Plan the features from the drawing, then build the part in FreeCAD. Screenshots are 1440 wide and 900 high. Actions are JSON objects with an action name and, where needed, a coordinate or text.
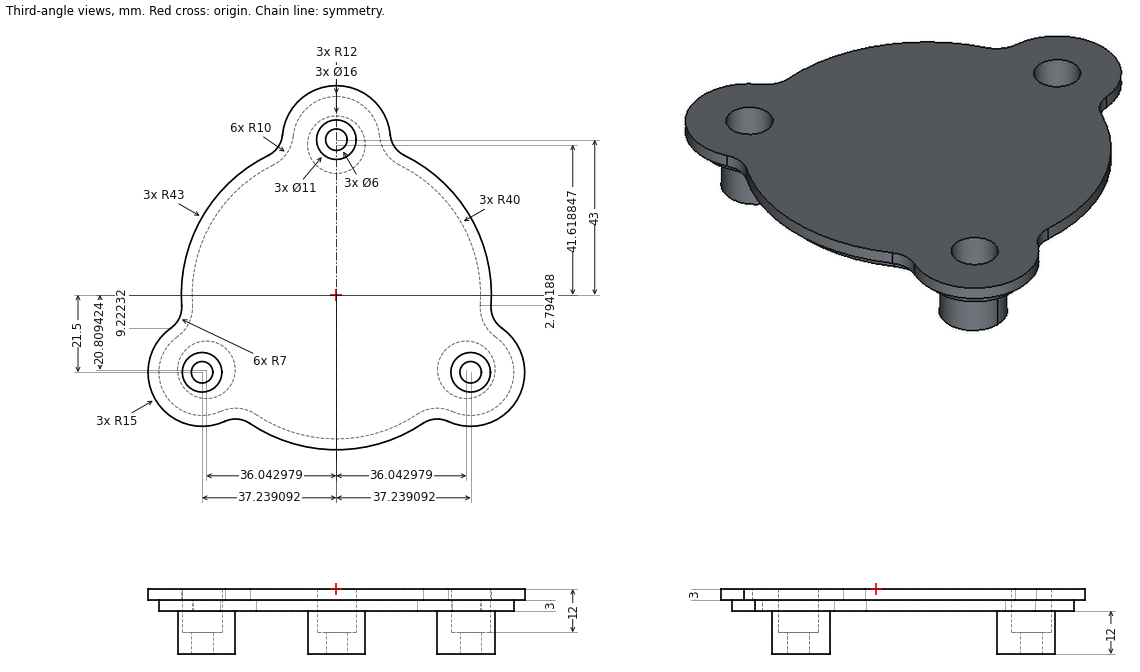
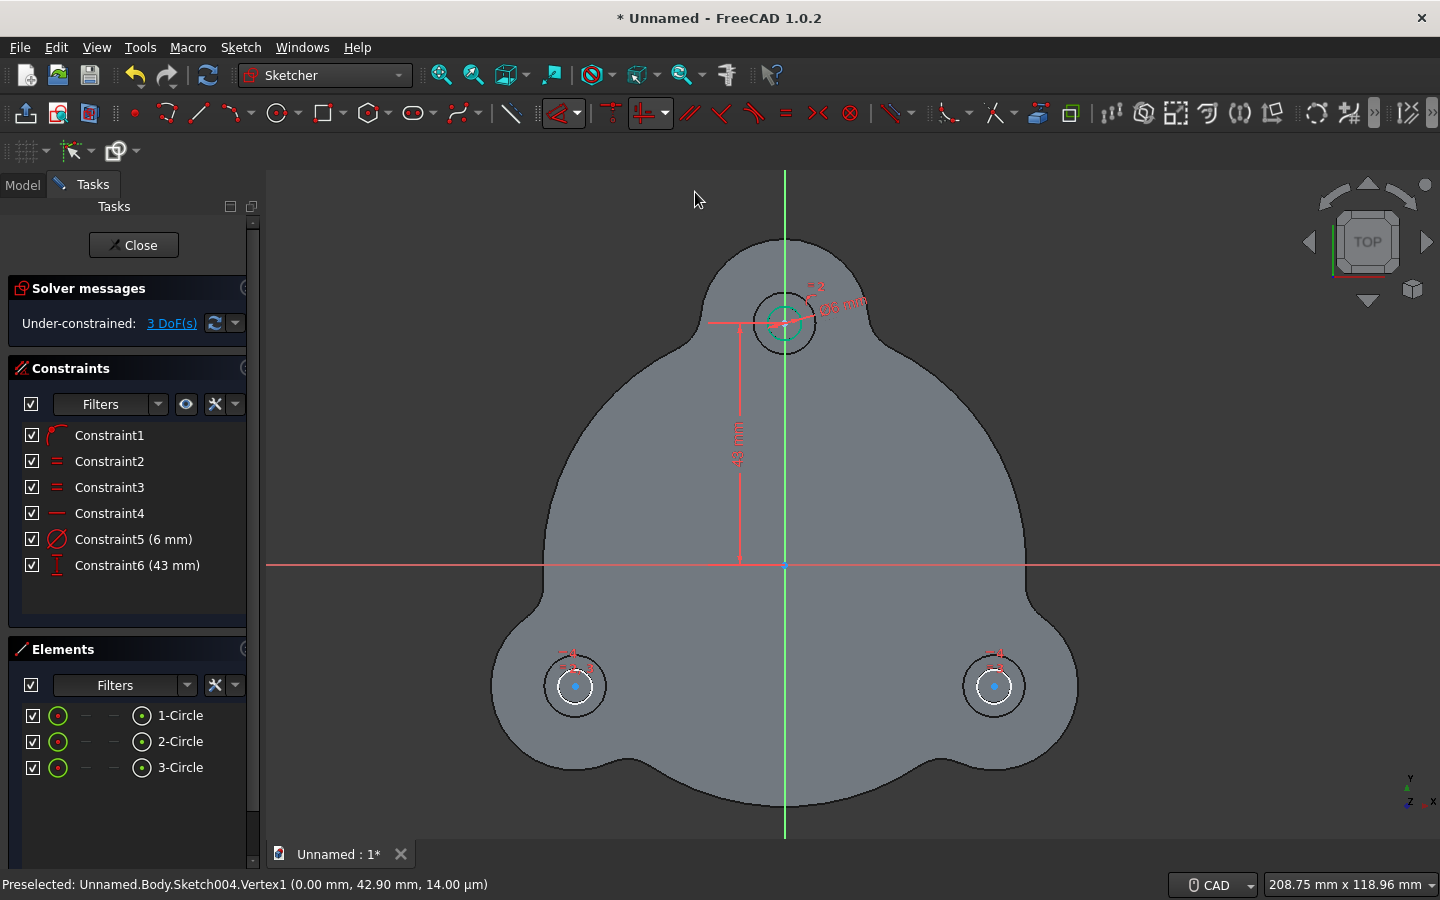
{"action": "left_click", "coordinate": [575, 687]}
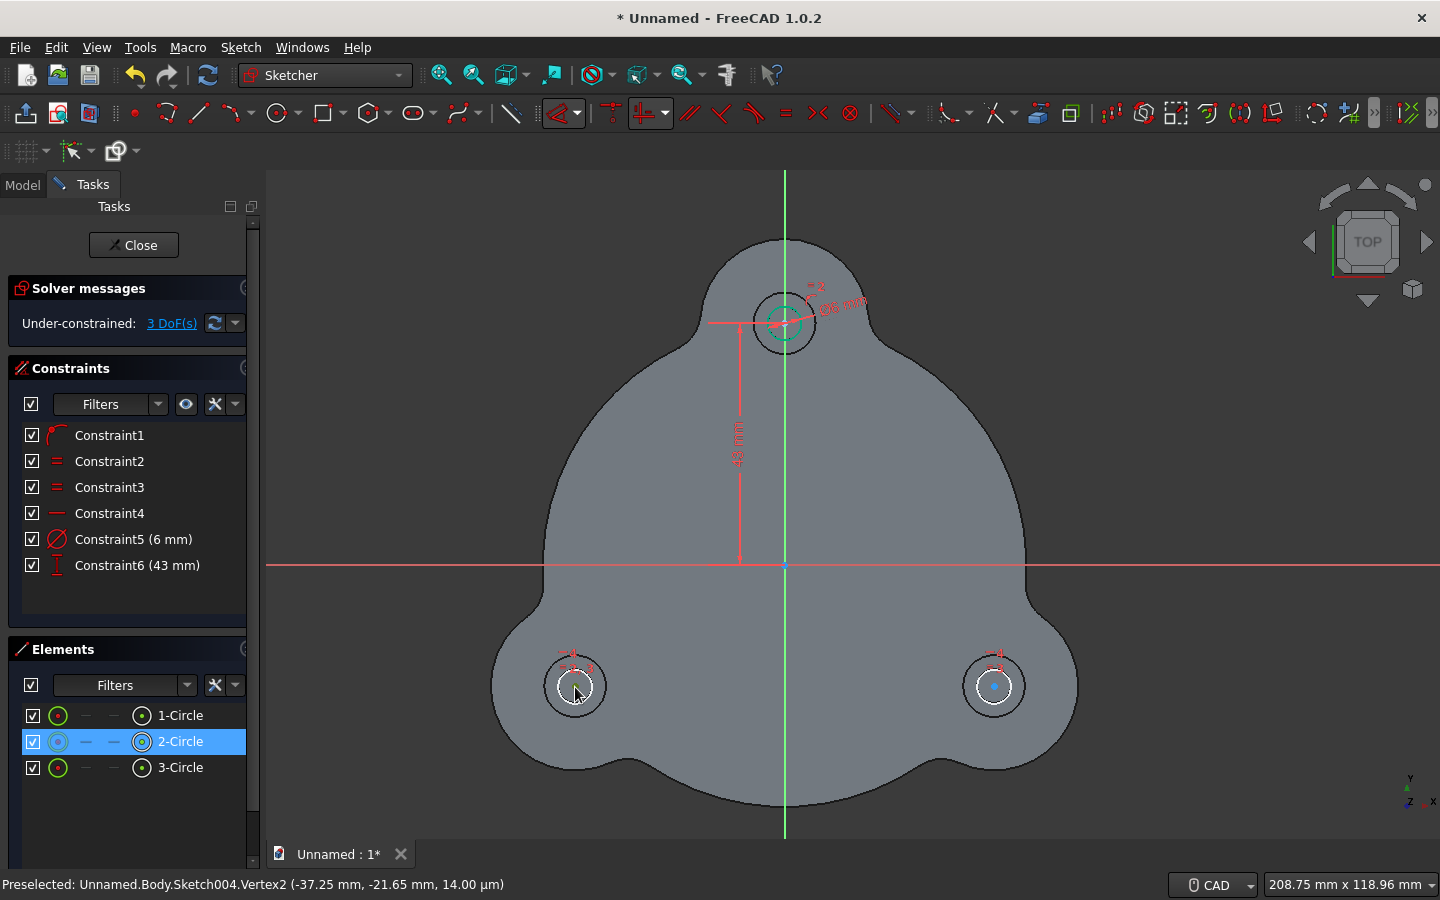
{"action": "left_click", "coordinate": [580, 114]}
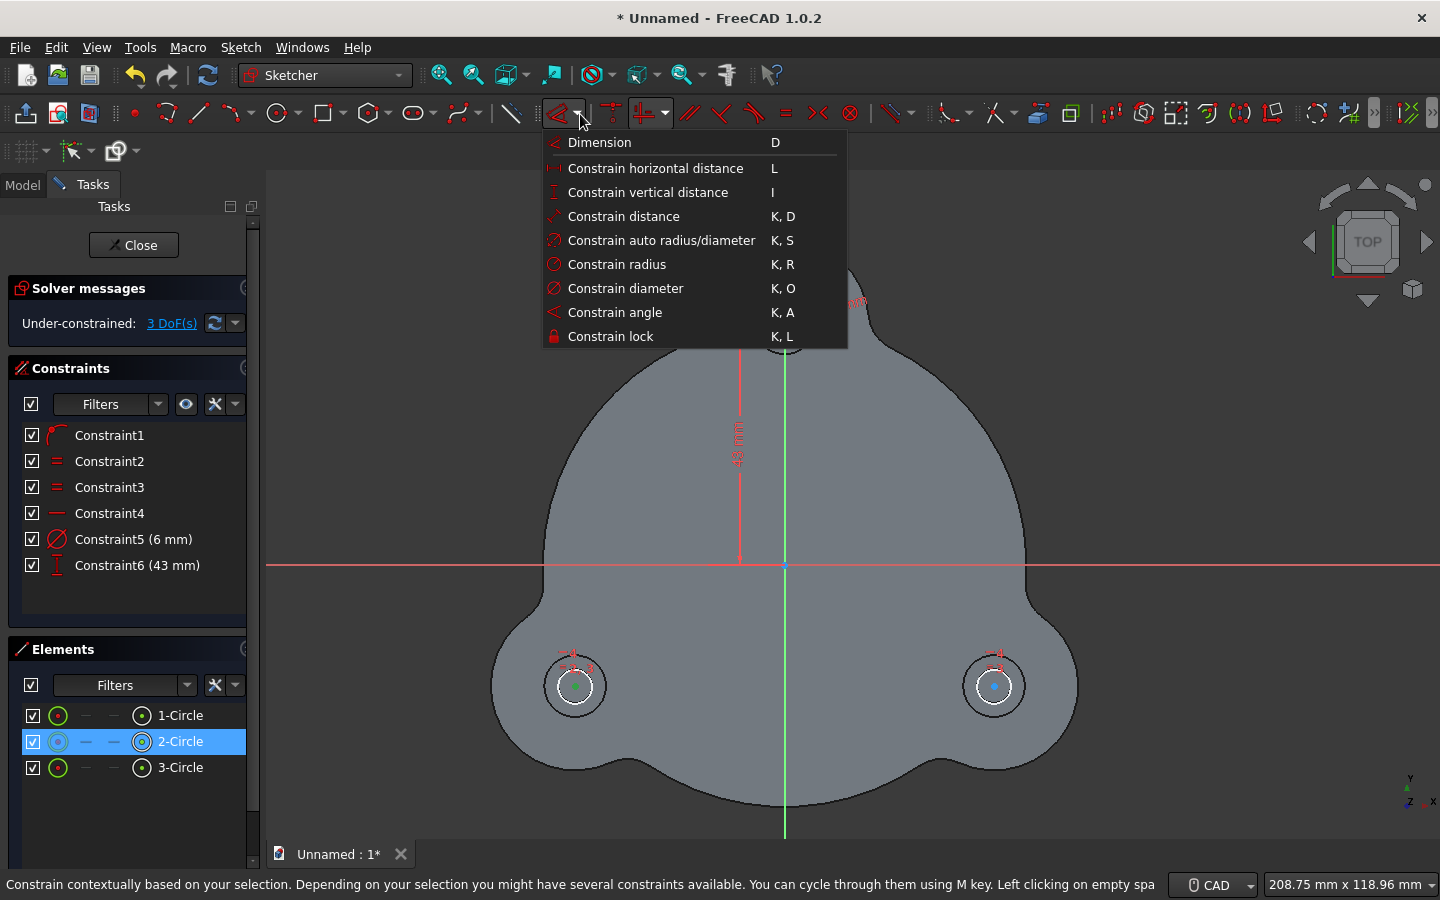
{"action": "left_click", "coordinate": [695, 192]}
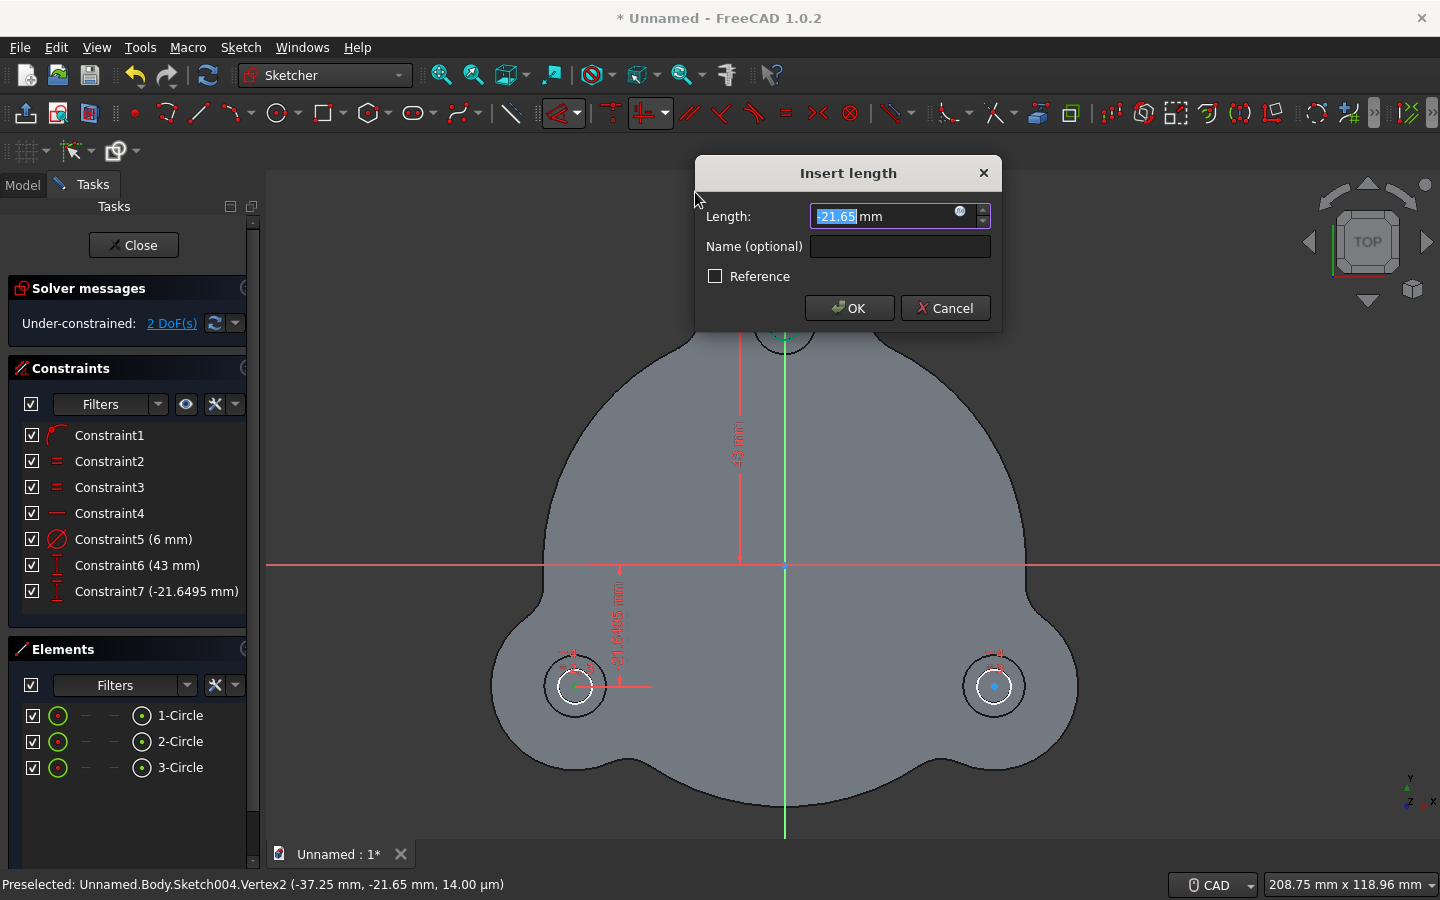
{"action": "type", "text": "-21.5"}
{"action": "key", "text": "Return"}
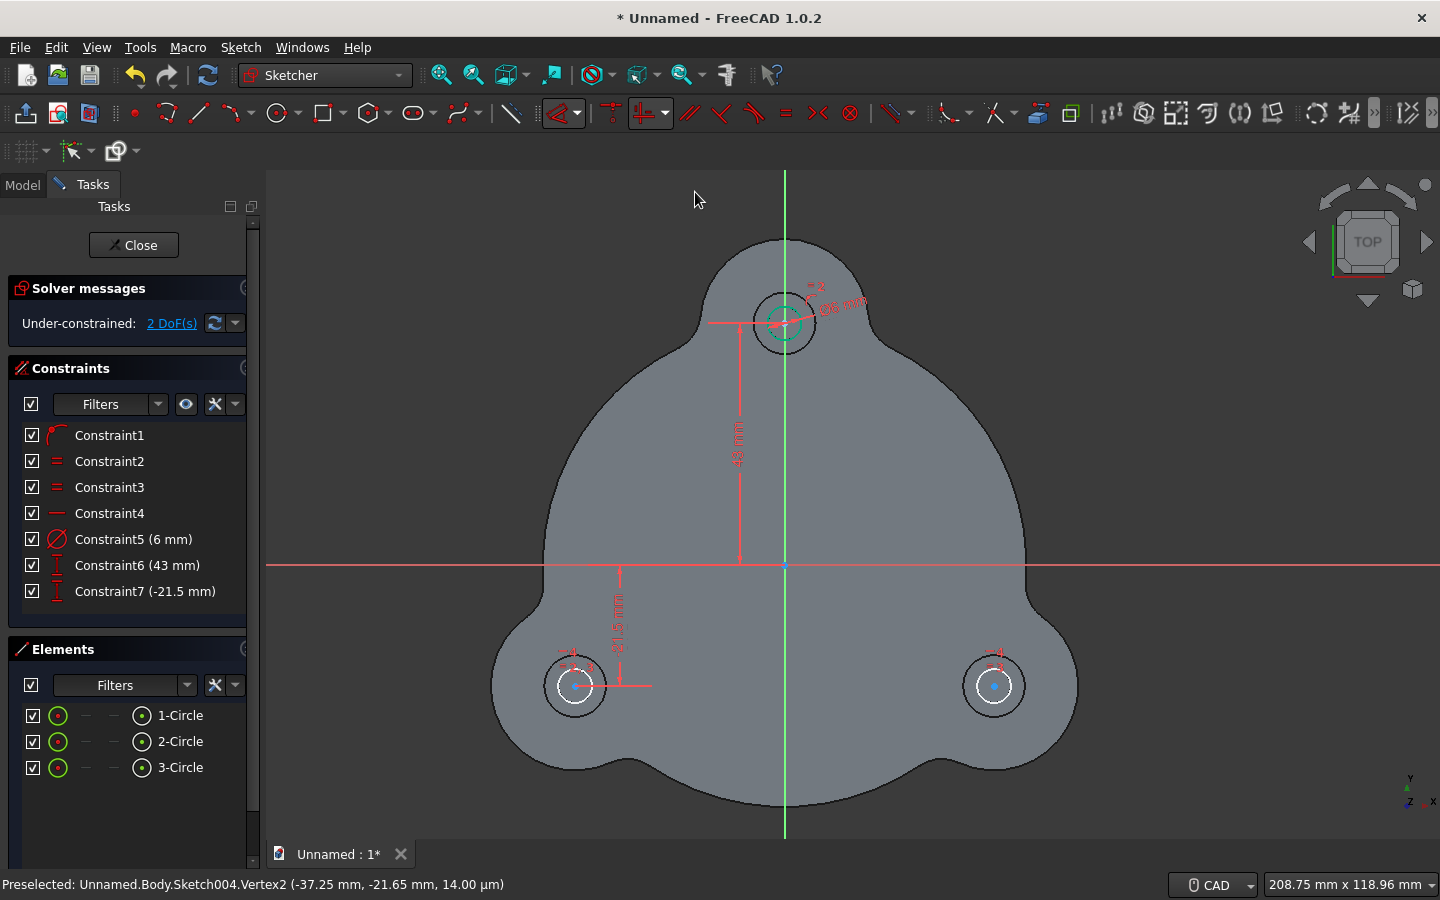
{"action": "left_click", "coordinate": [575, 686]}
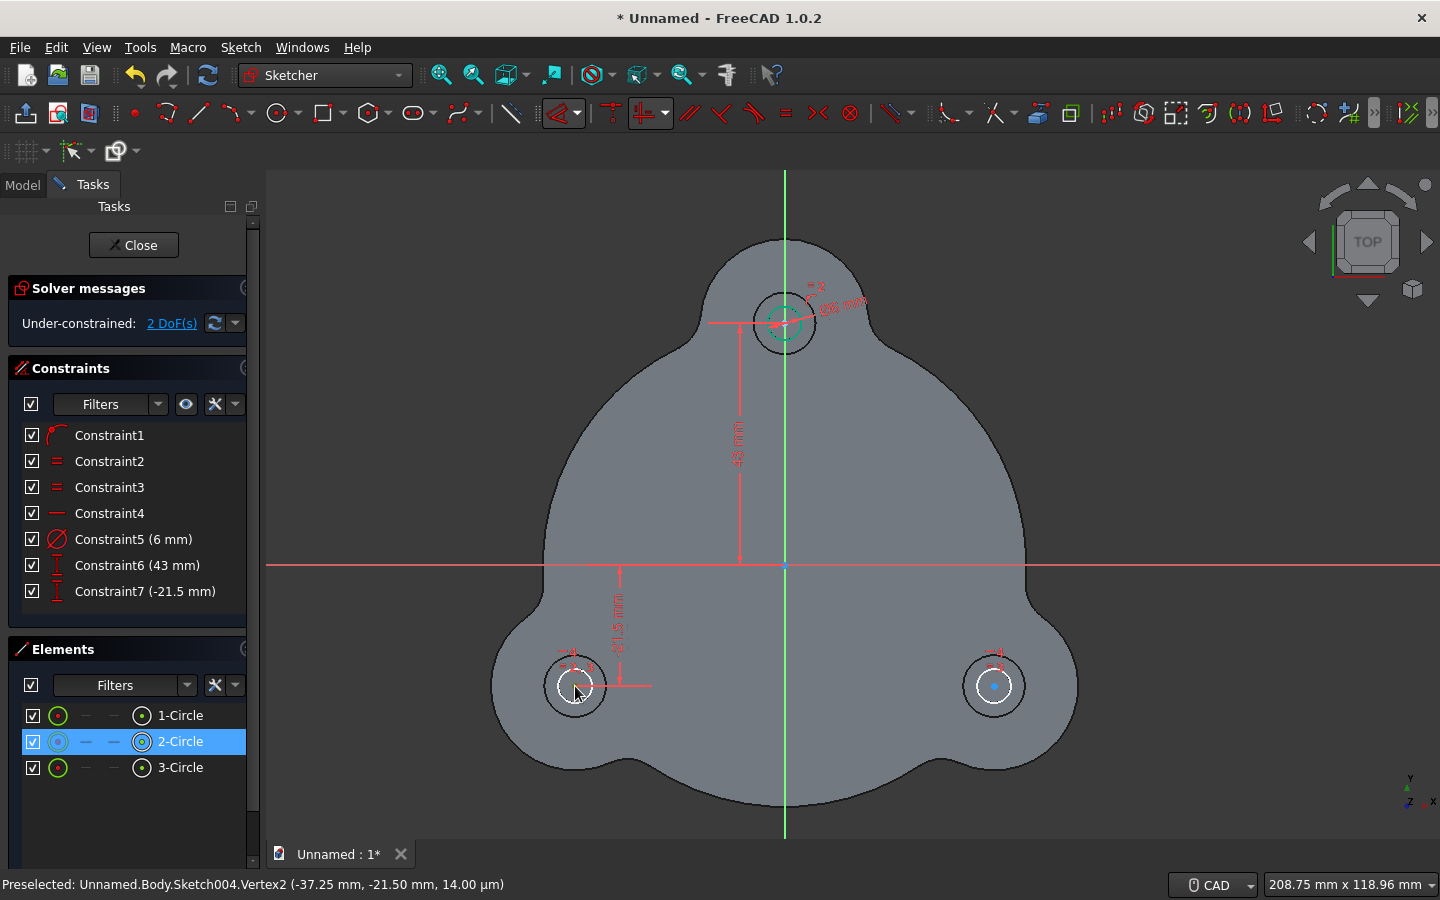
{"action": "left_click", "coordinate": [580, 114]}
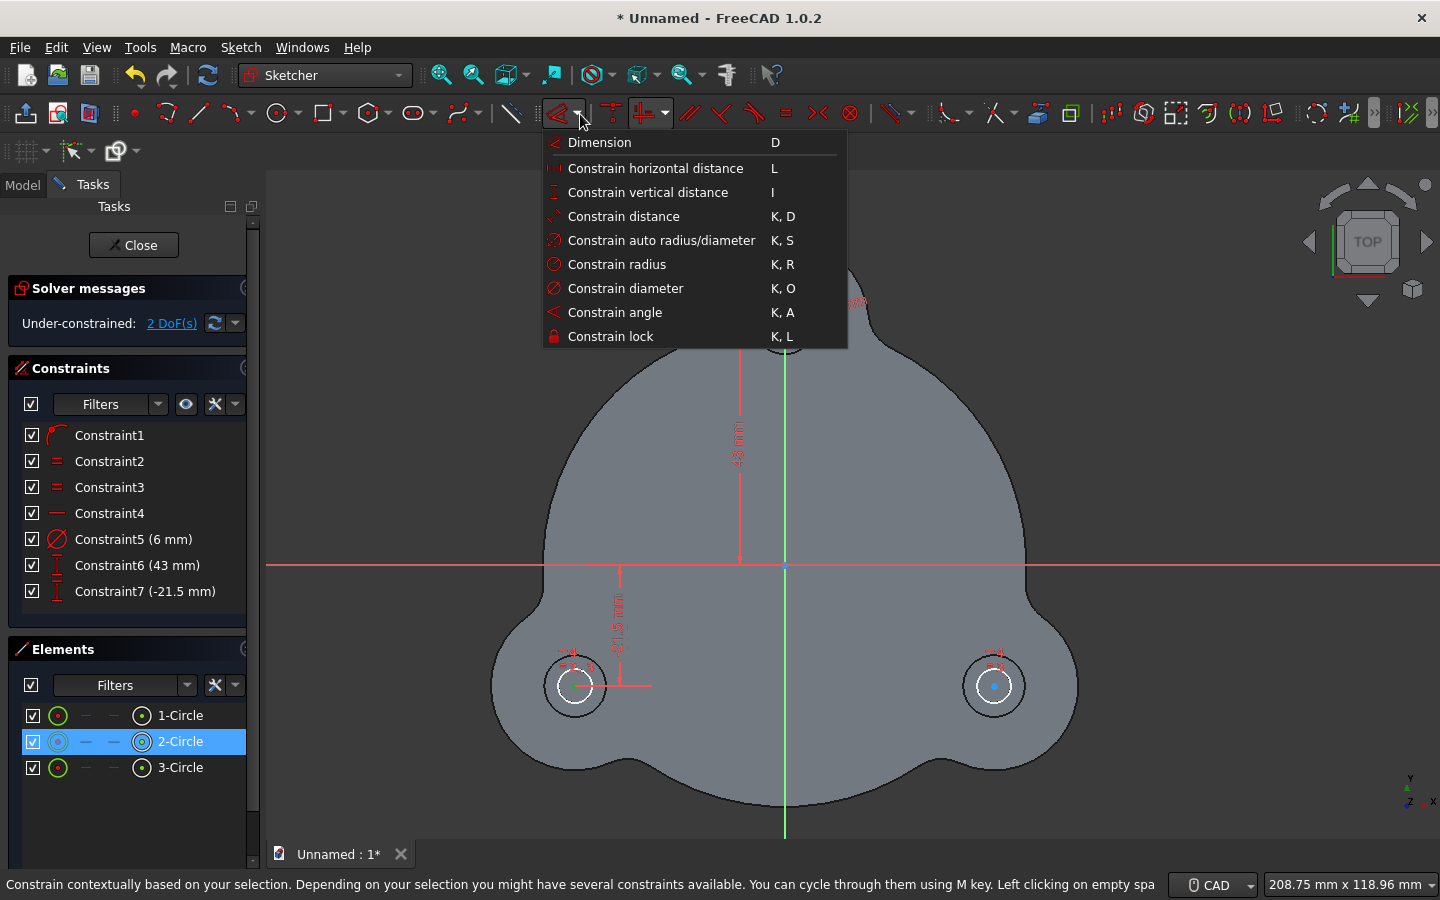
{"action": "left_click", "coordinate": [695, 168]}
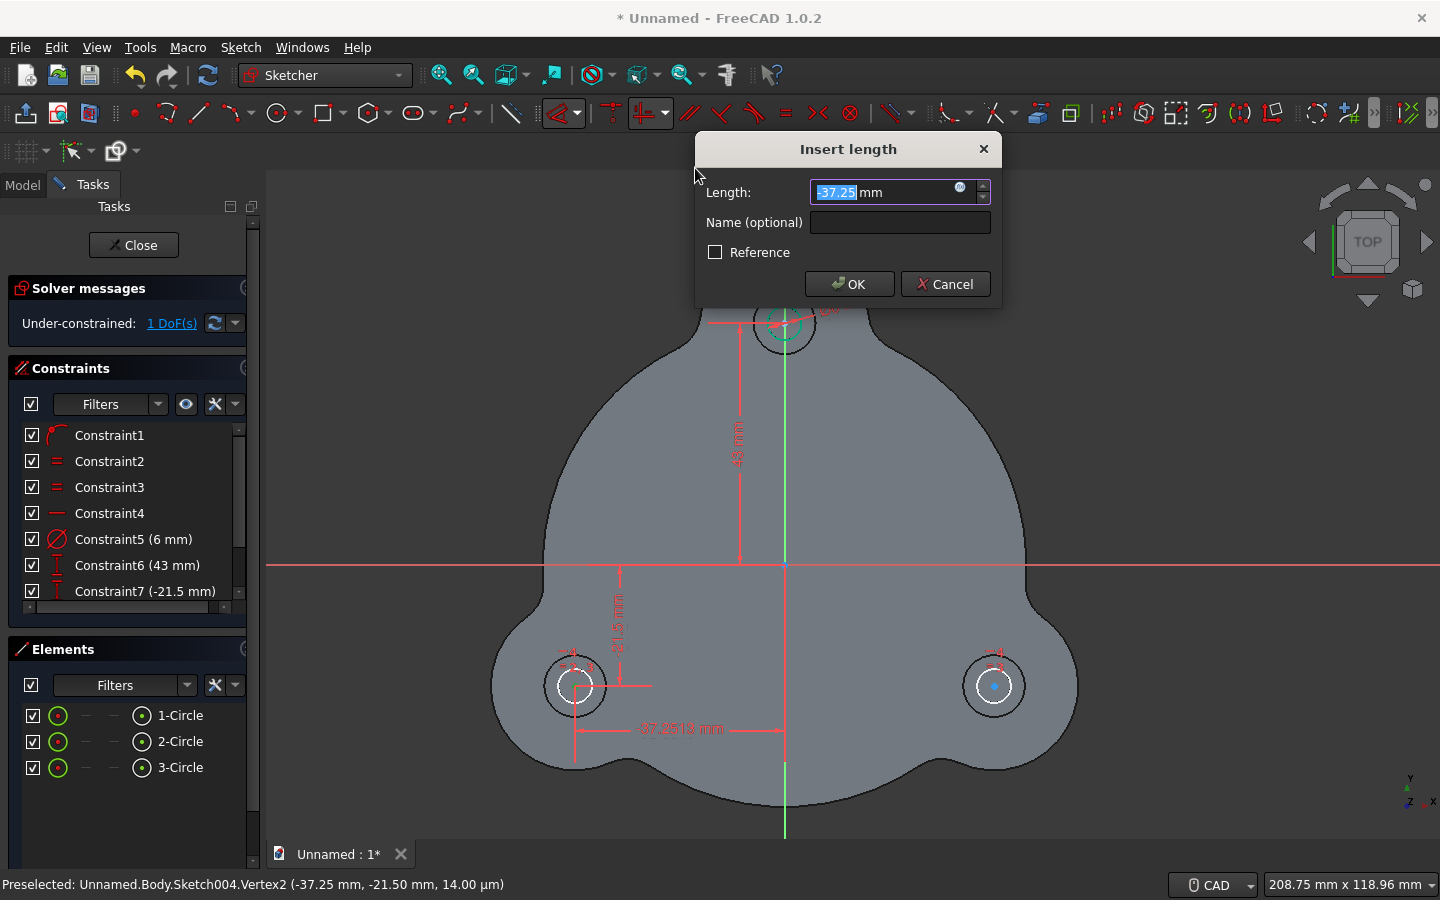
{"action": "type", "text": "-37.239092"}
{"action": "key", "text": "Return"}